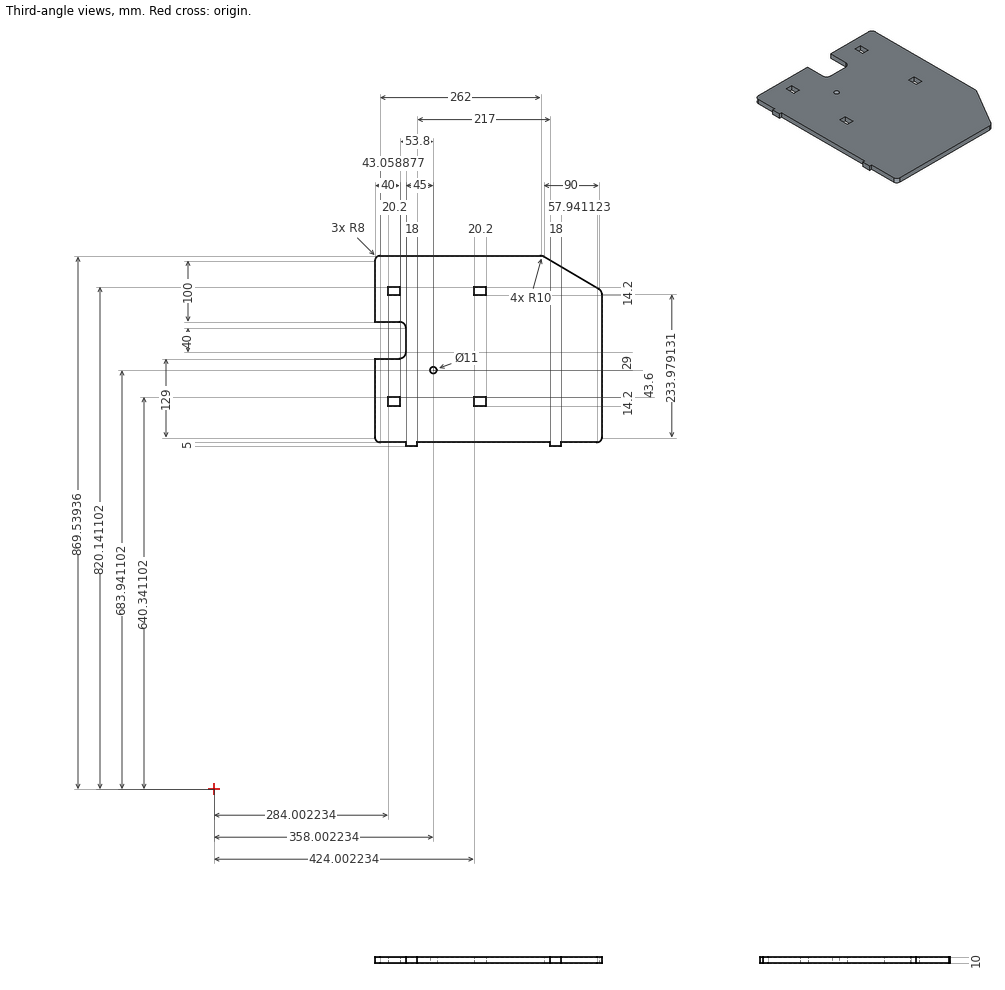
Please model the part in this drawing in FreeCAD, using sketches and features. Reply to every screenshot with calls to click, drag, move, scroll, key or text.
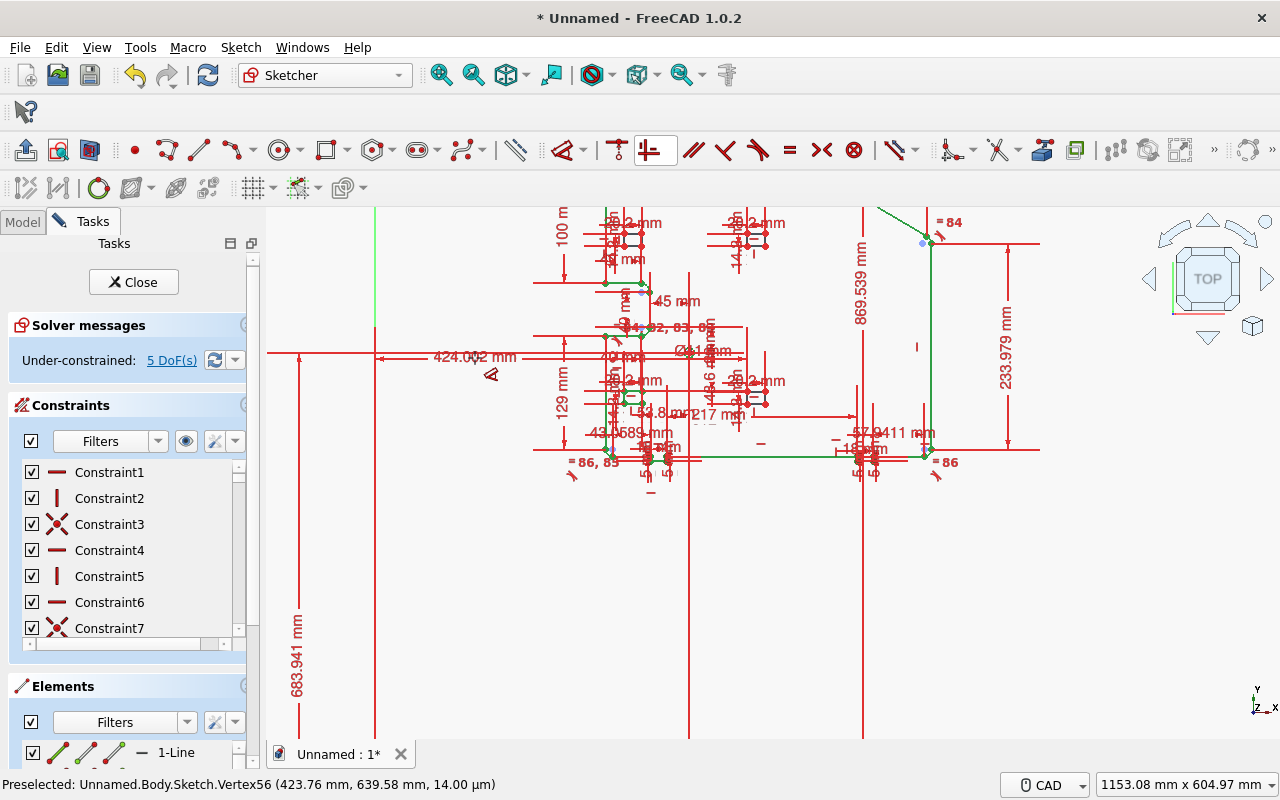
click(747, 392)
click(341, 551)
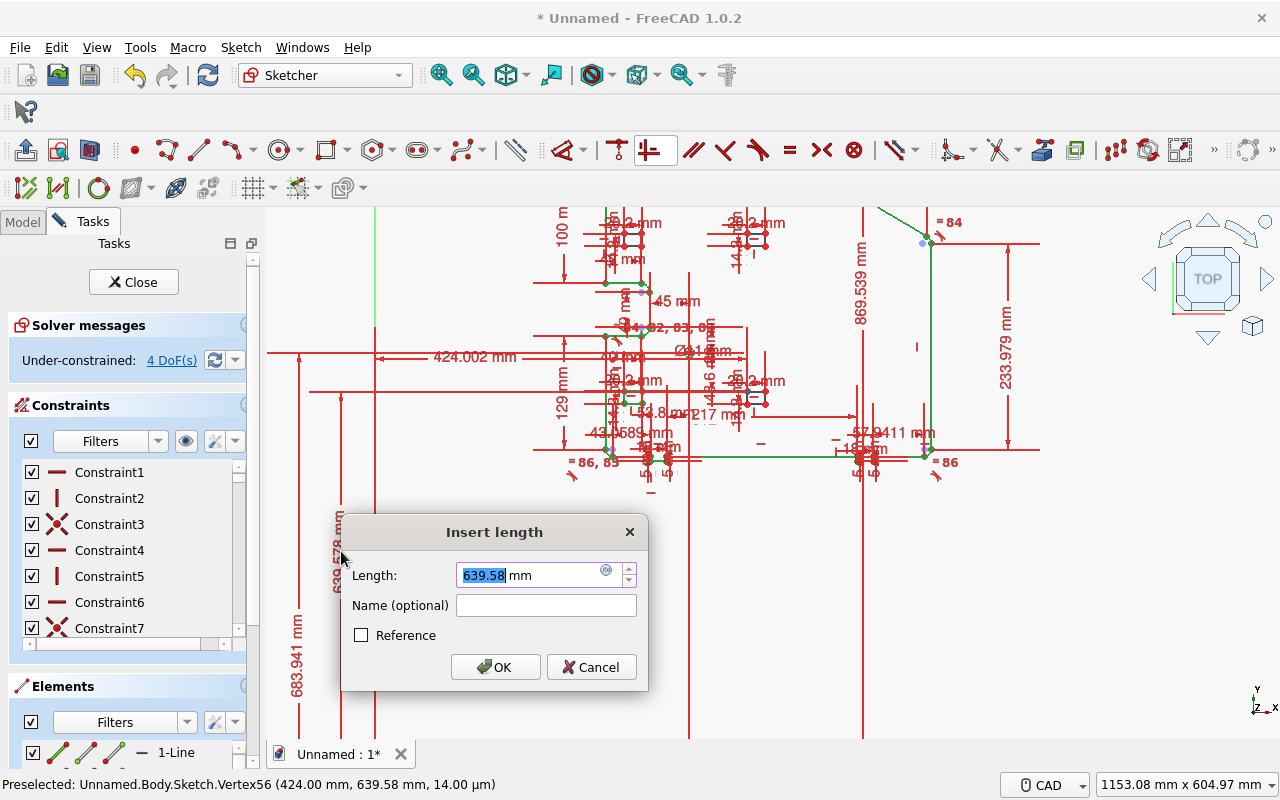
text(640.341102)
key(Return)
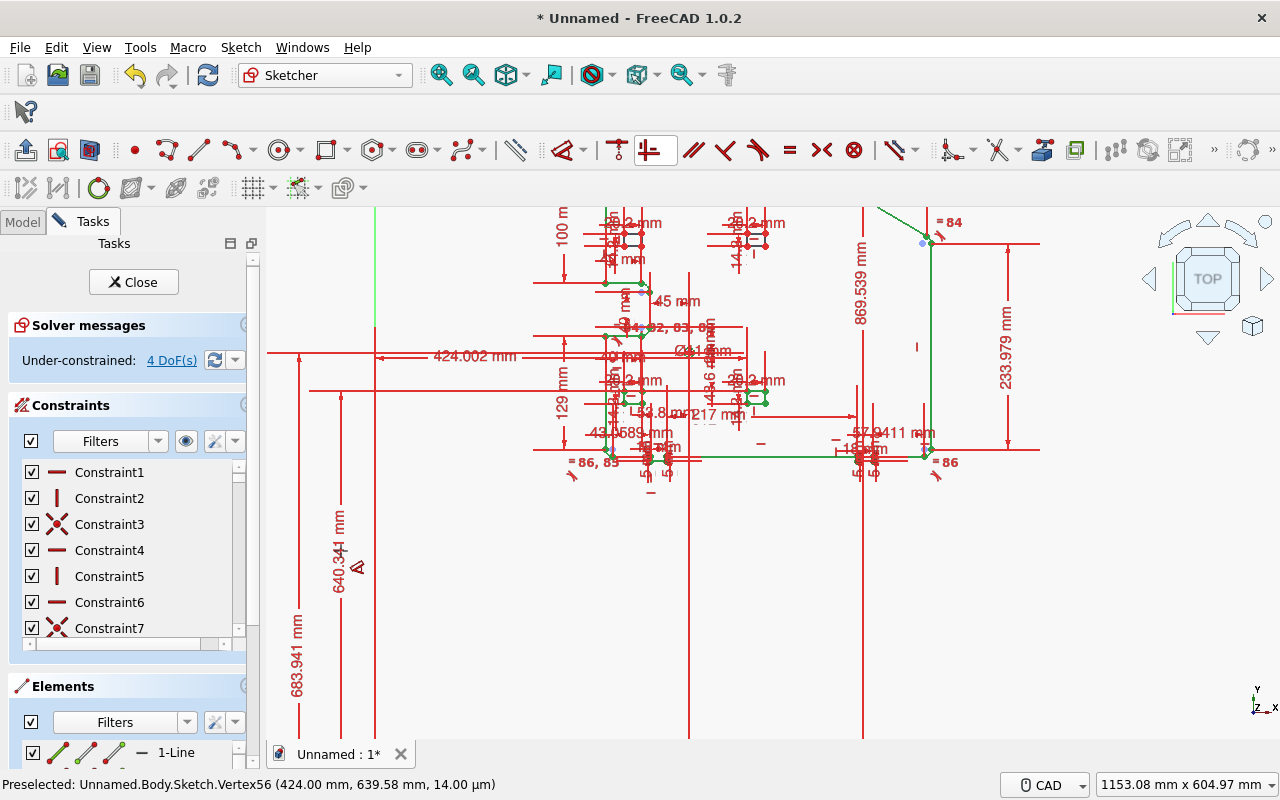
scroll(747, 393, down, 4)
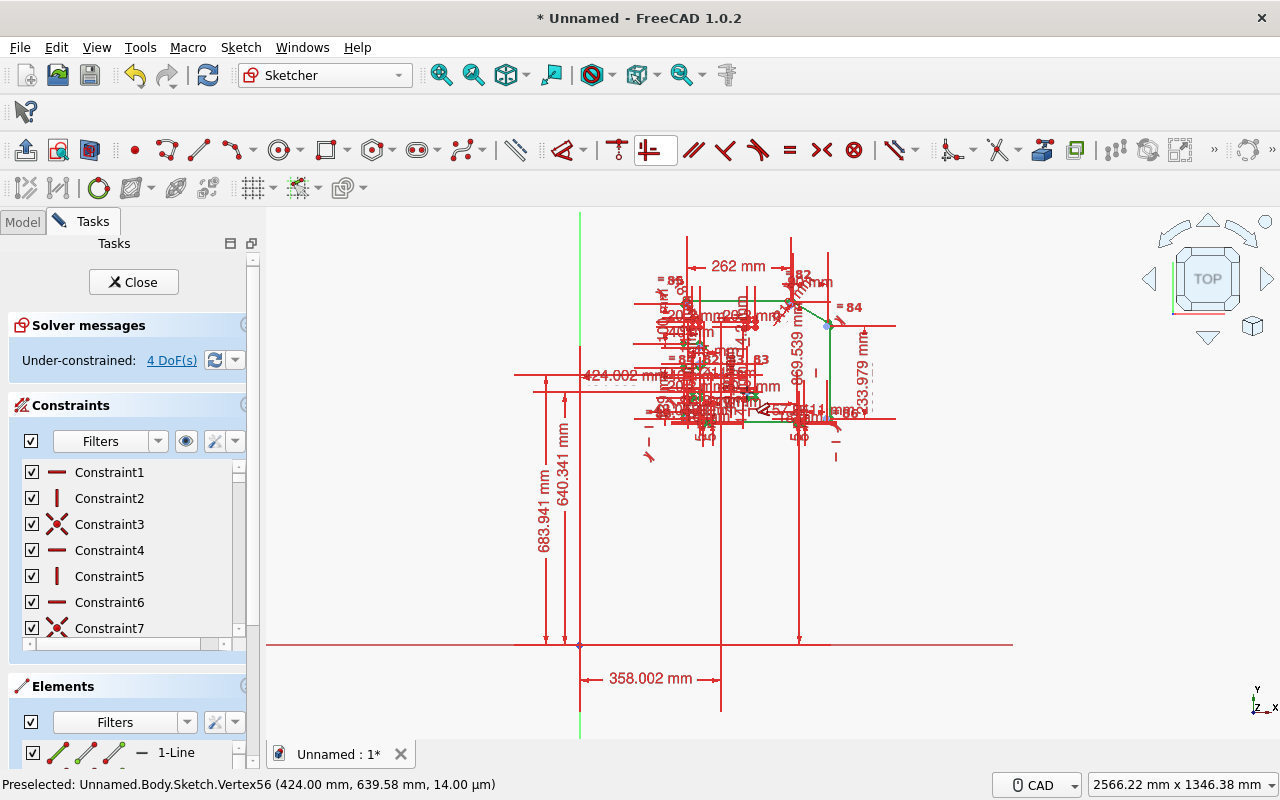
scroll(747, 322, up, 4)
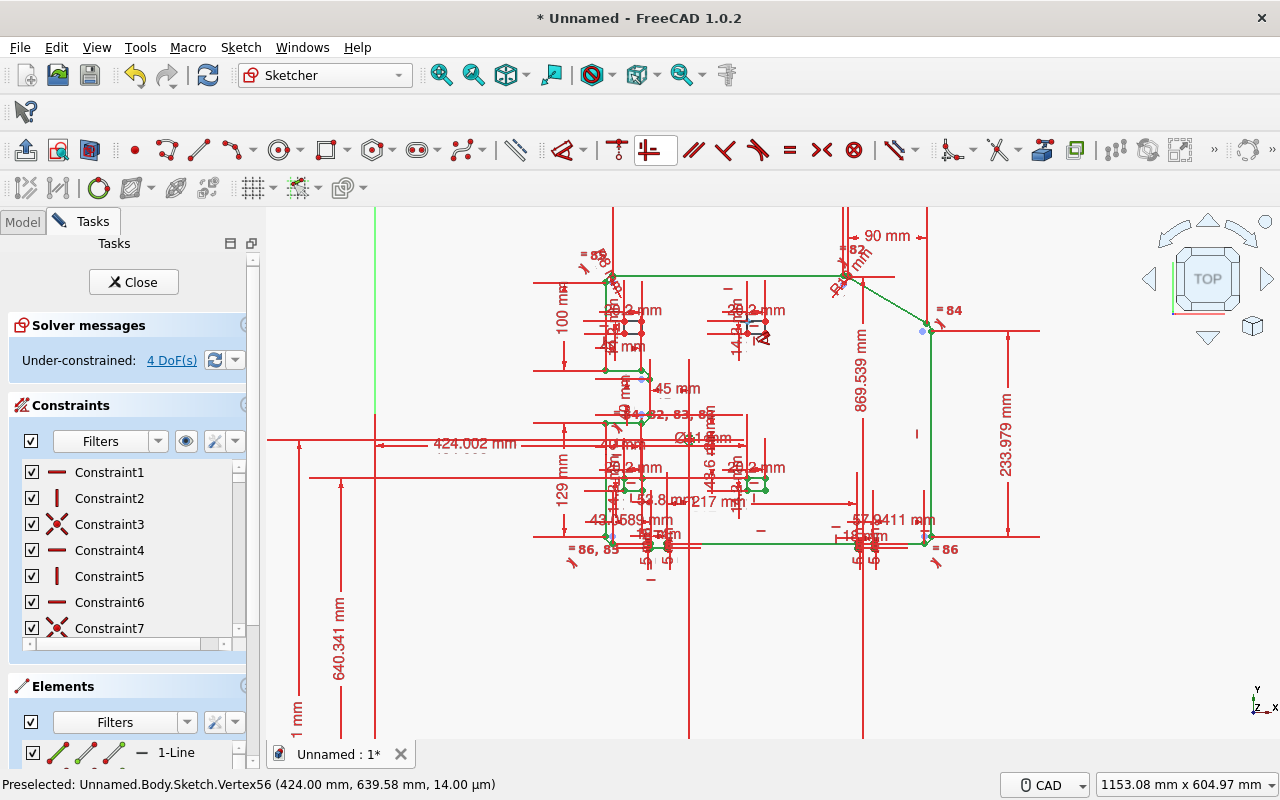
click(747, 321)
click(475, 287)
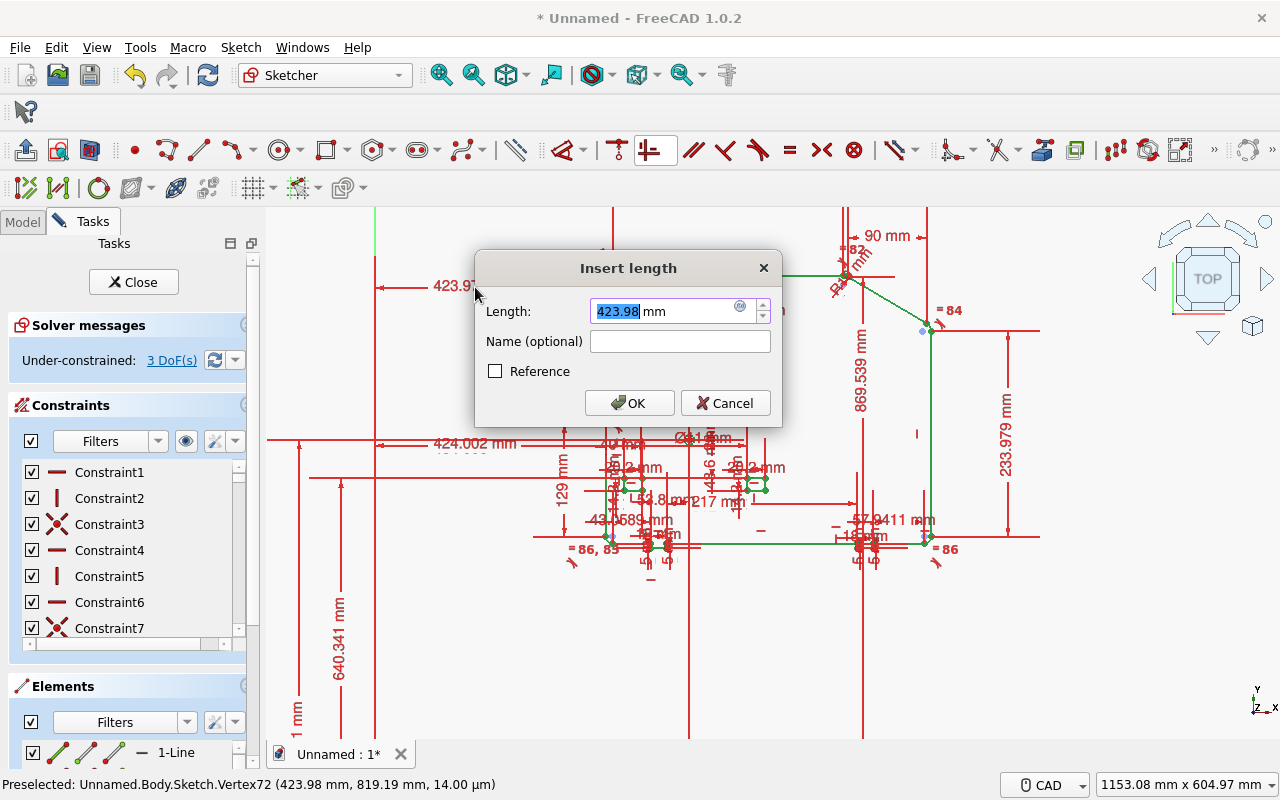
text(424.002234)
key(Return)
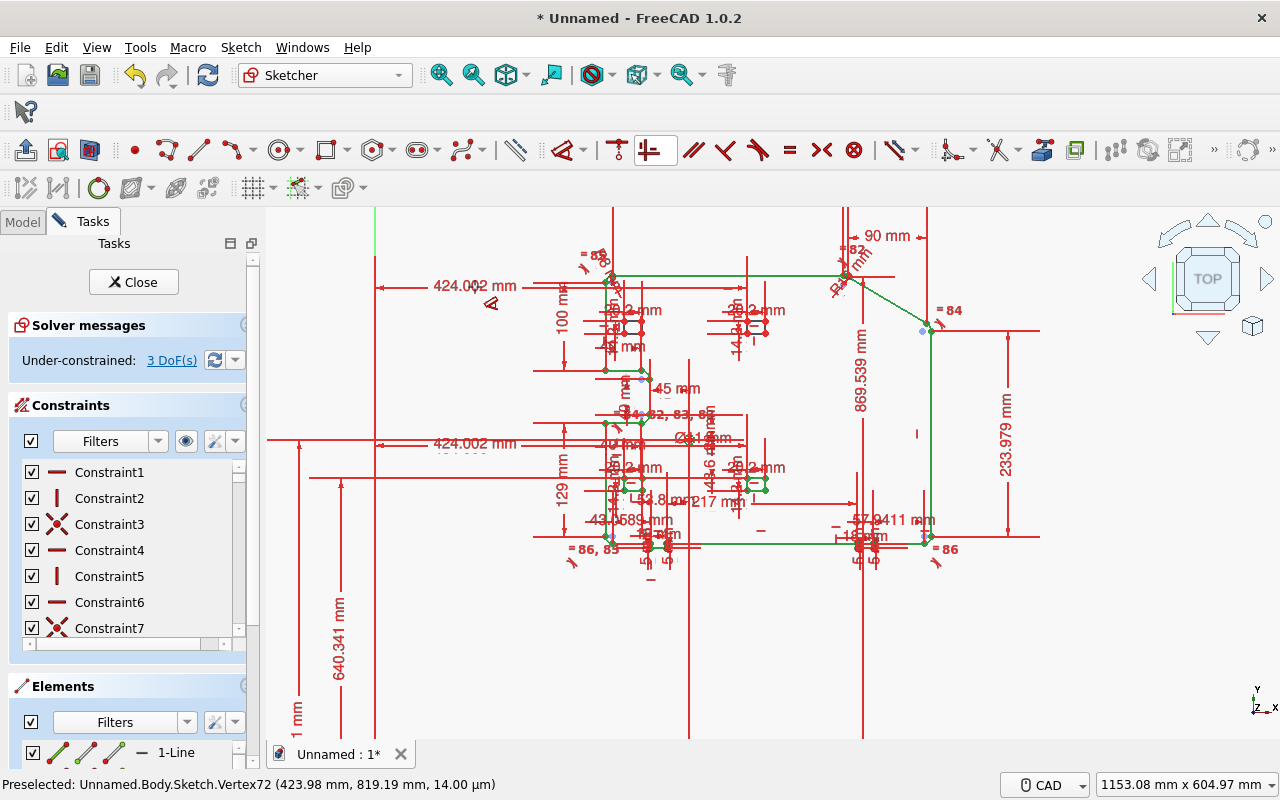
click(747, 321)
click(341, 516)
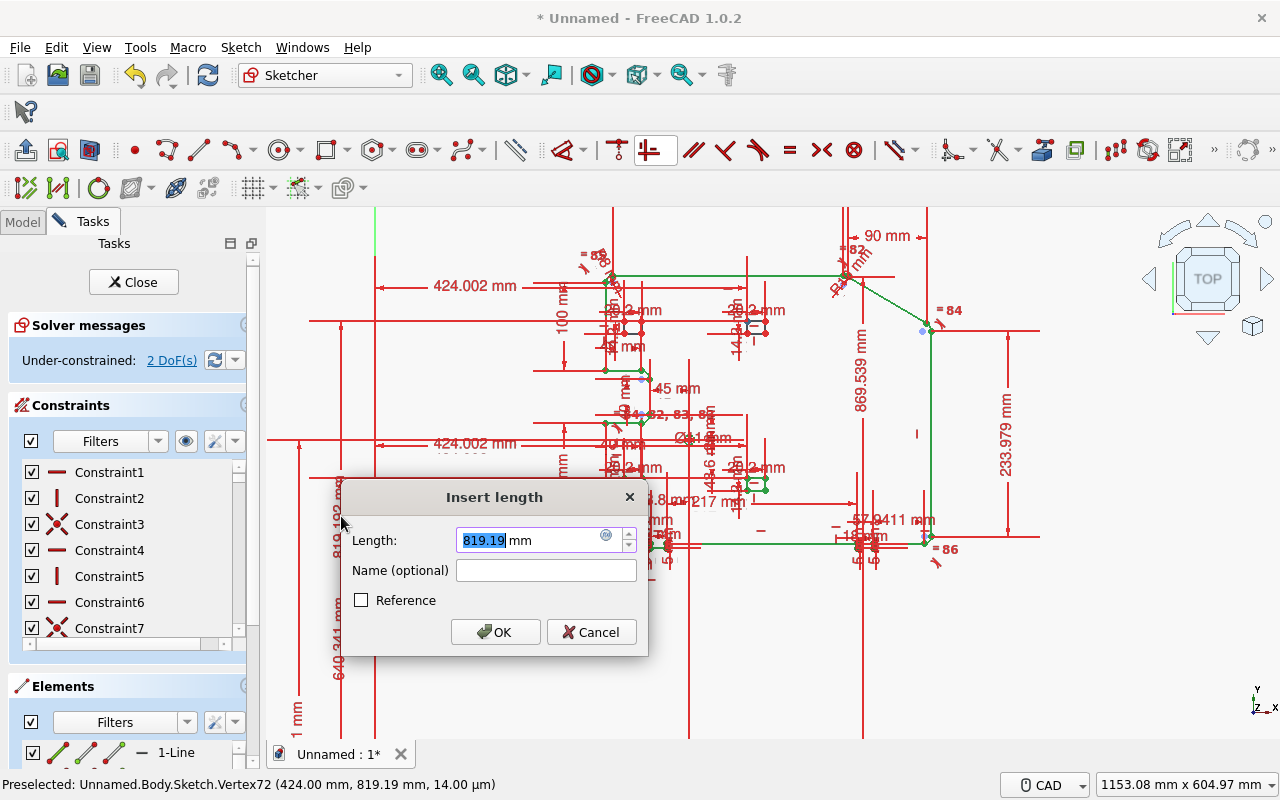
text(820.141102)
key(Return)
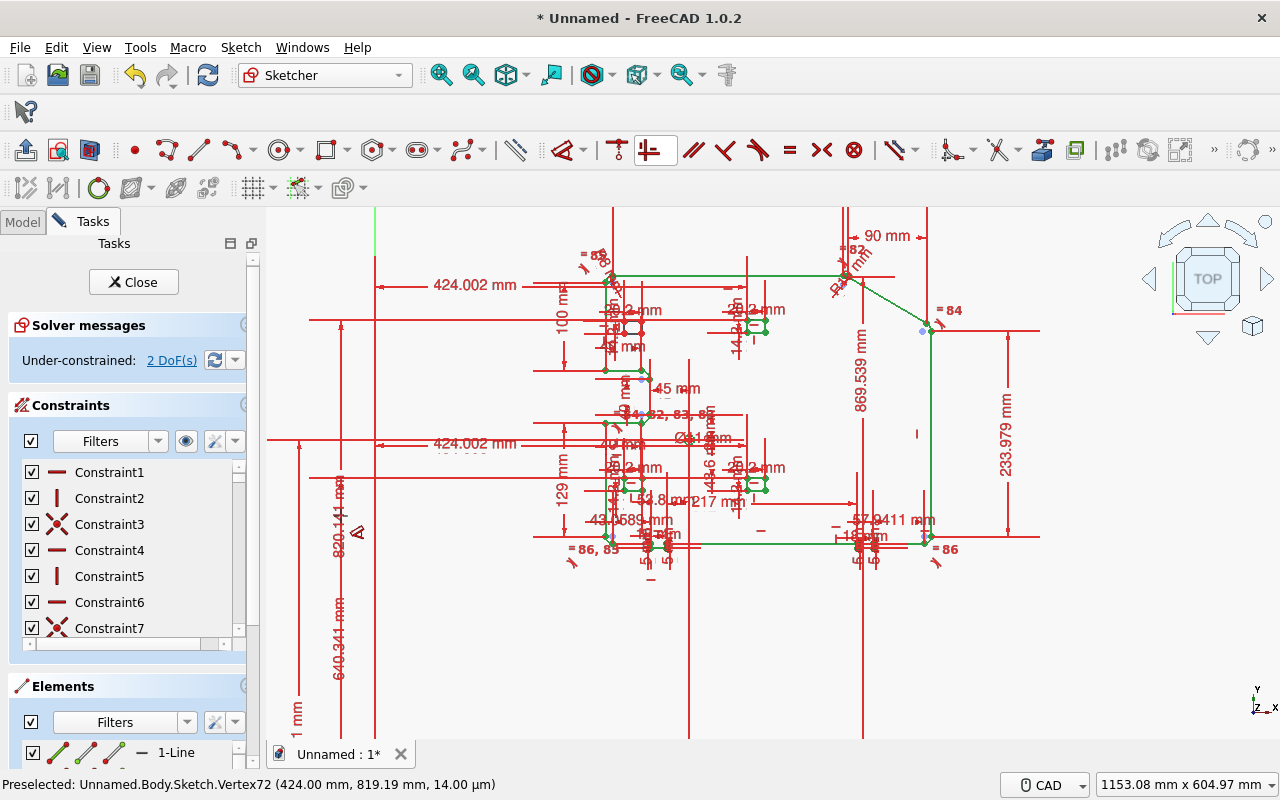
click(624, 321)
click(499, 263)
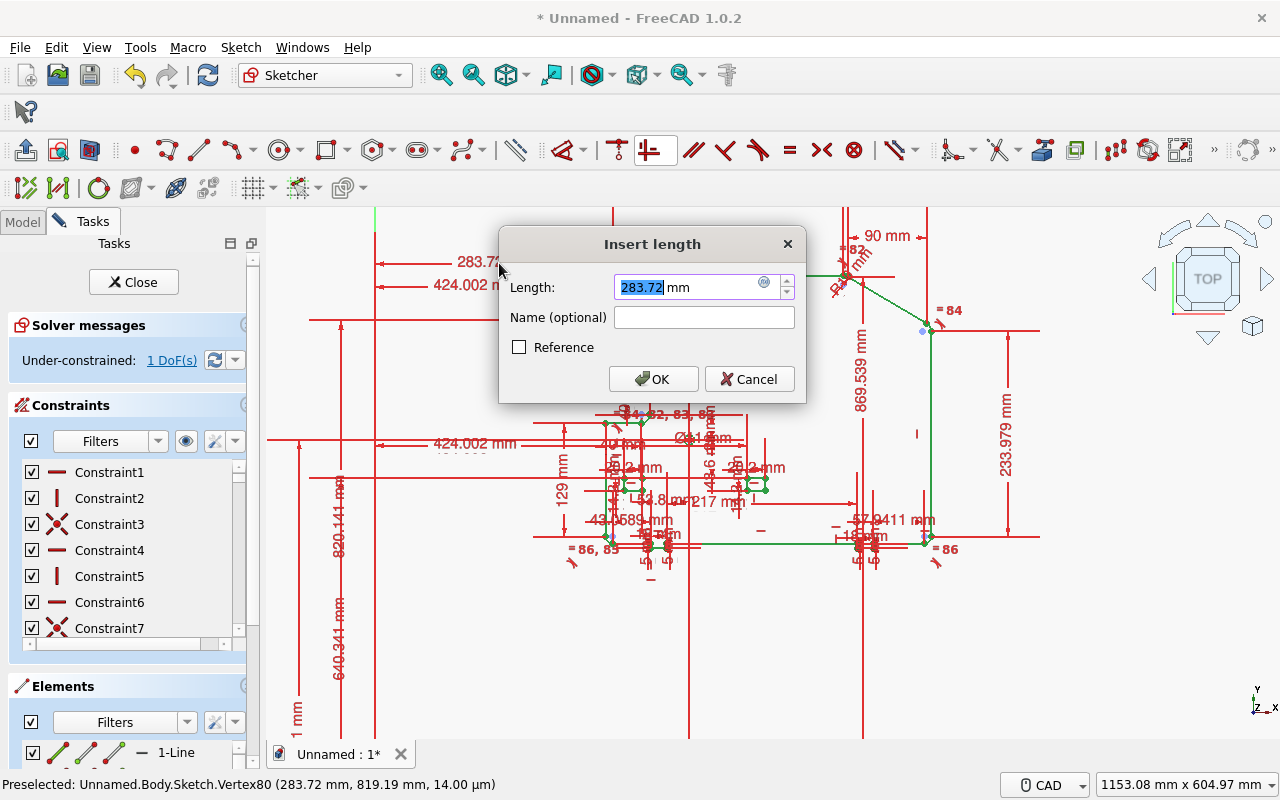
text(284.002234)
key(Return)